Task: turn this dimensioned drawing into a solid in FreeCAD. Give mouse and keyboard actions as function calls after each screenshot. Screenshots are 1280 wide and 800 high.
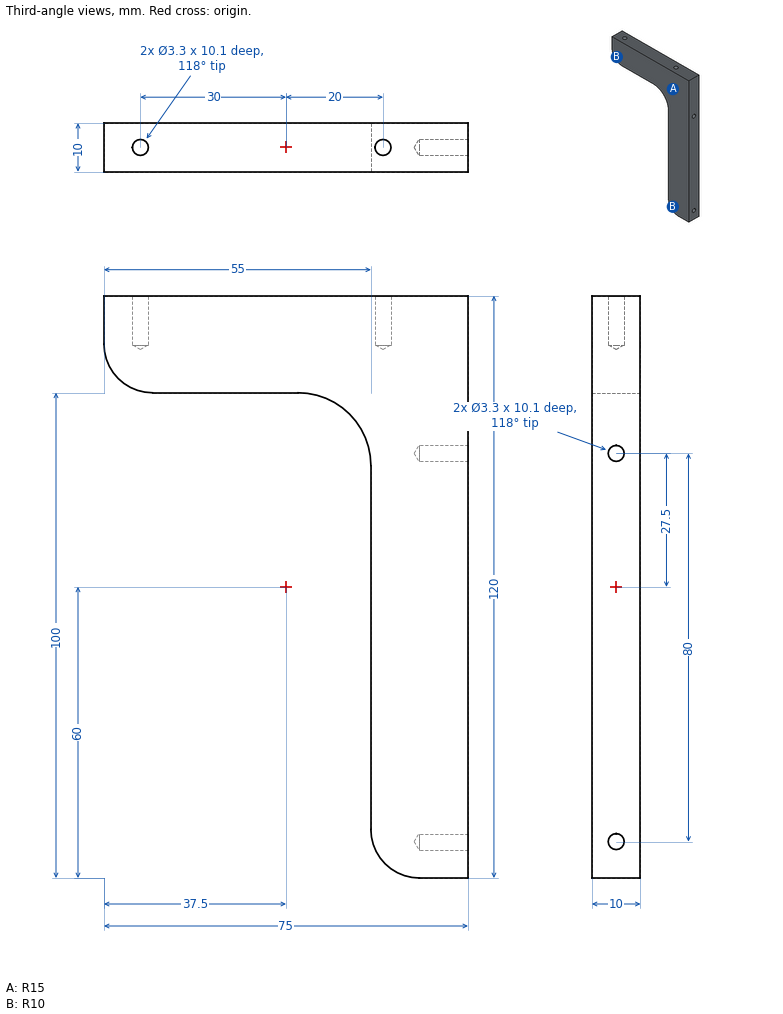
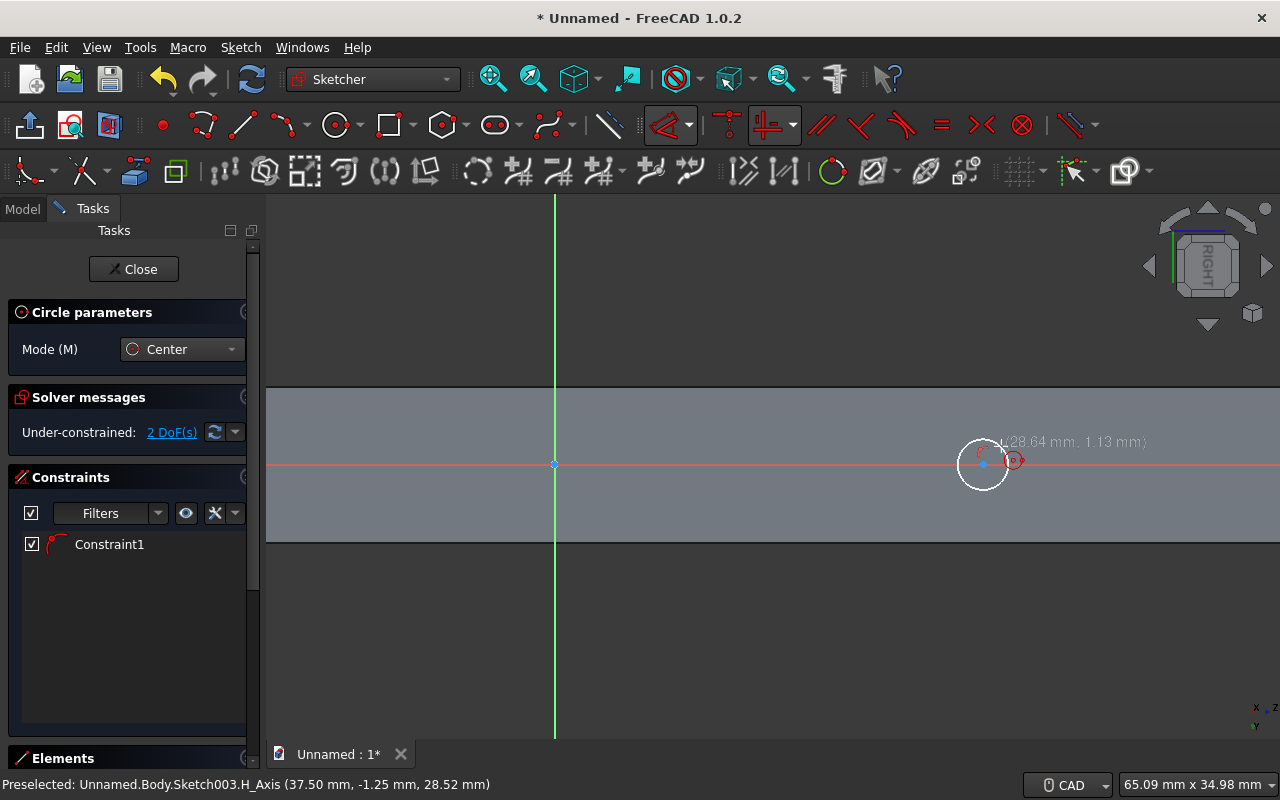
scroll(986, 468, down, 4)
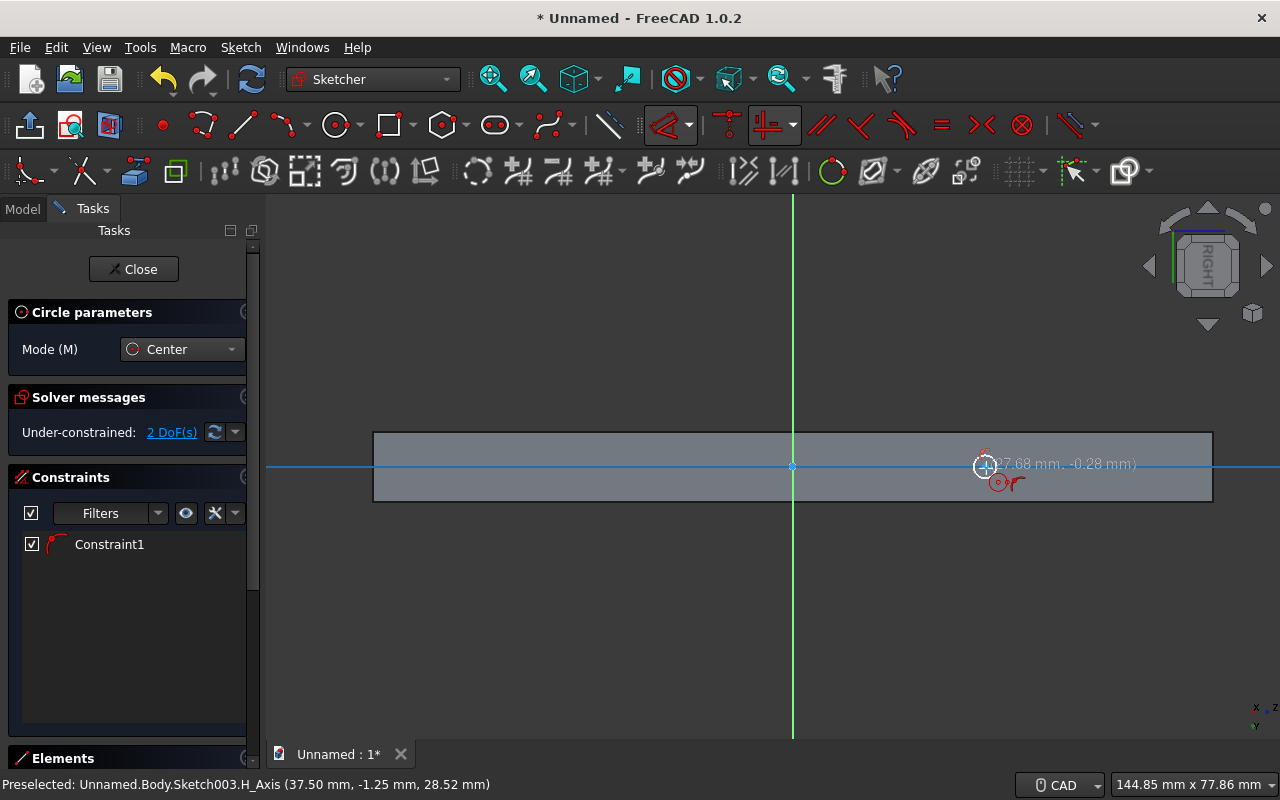
scroll(425, 467, up, 4)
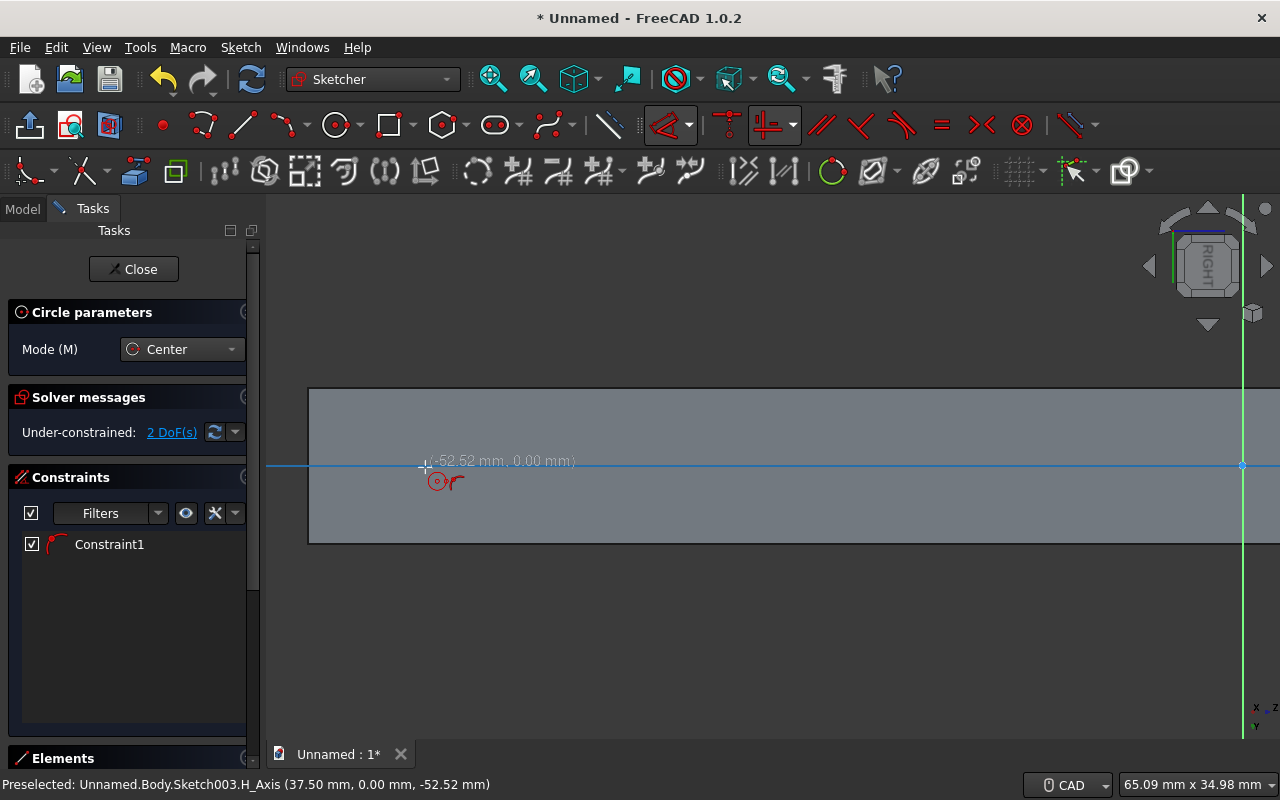
click(425, 466)
click(443, 448)
key(Escape)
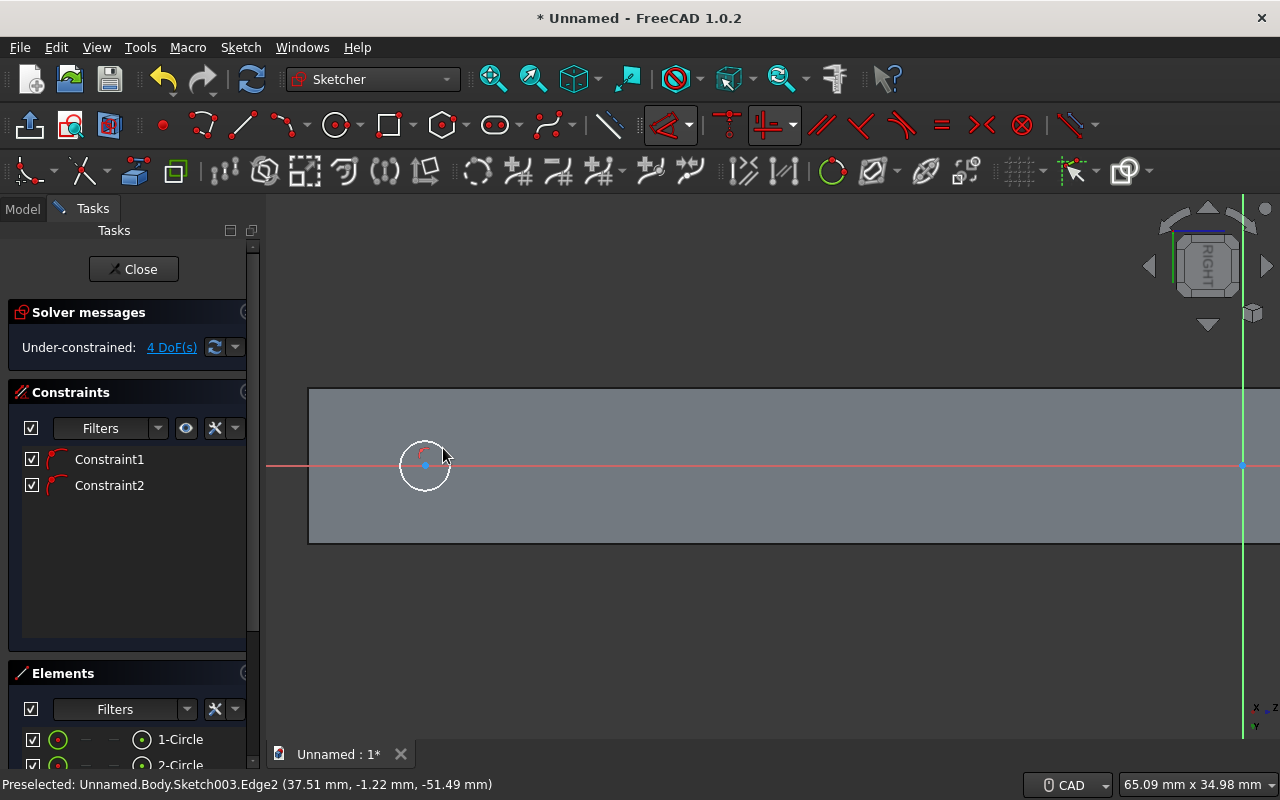
scroll(424, 467, down, 4)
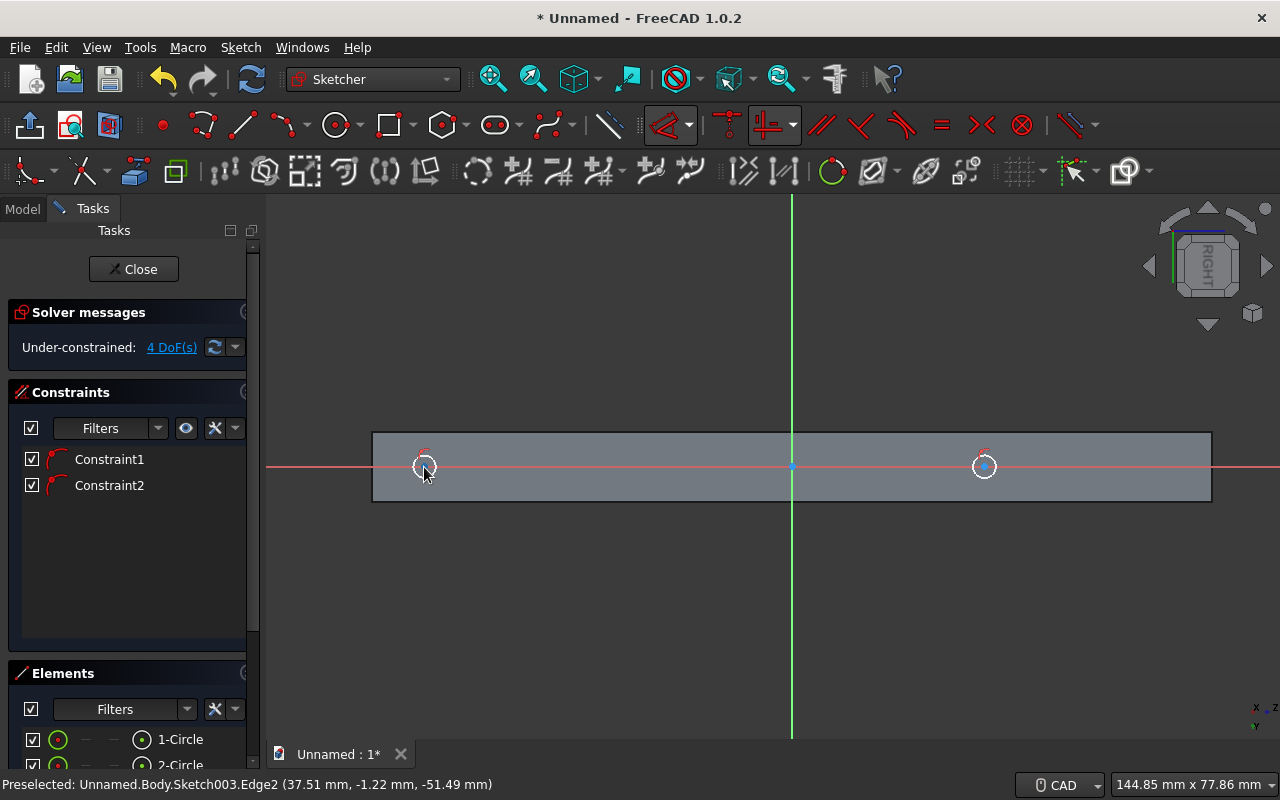
scroll(992, 459, up, 3)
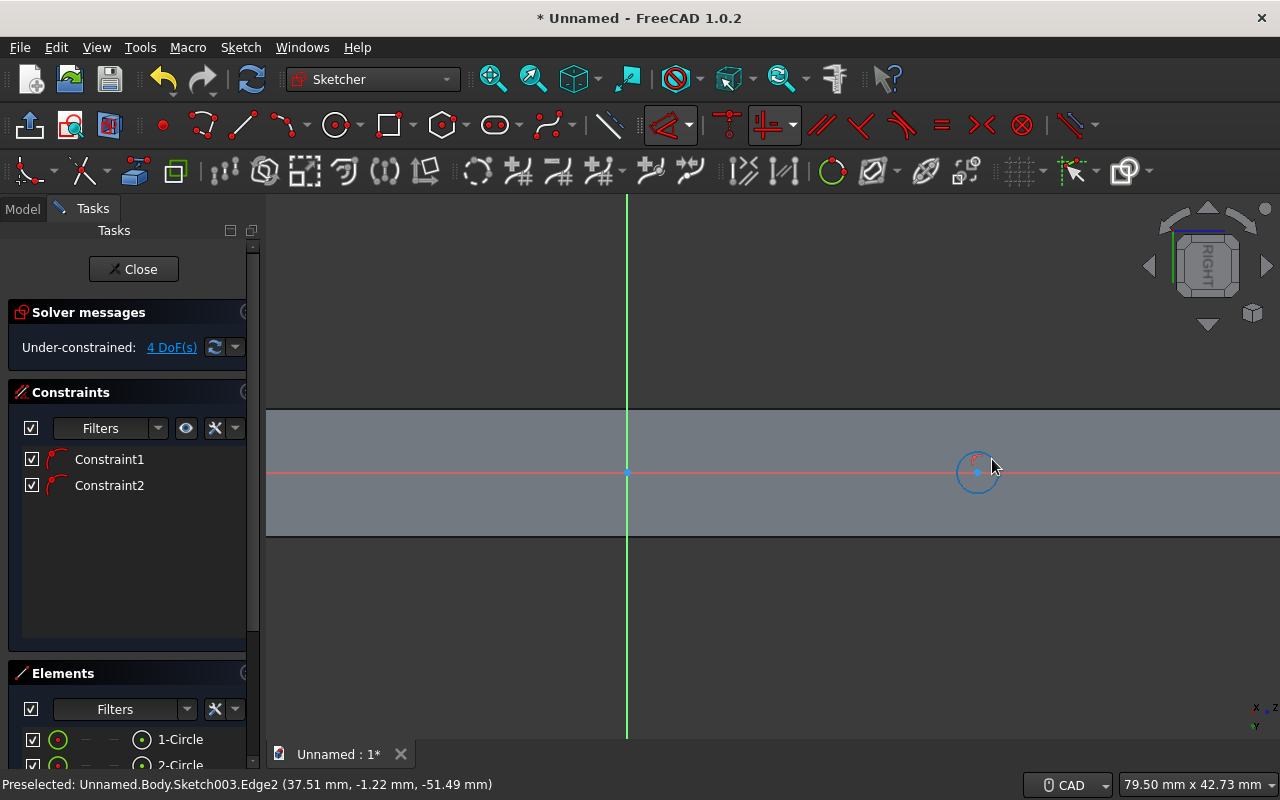
click(992, 458)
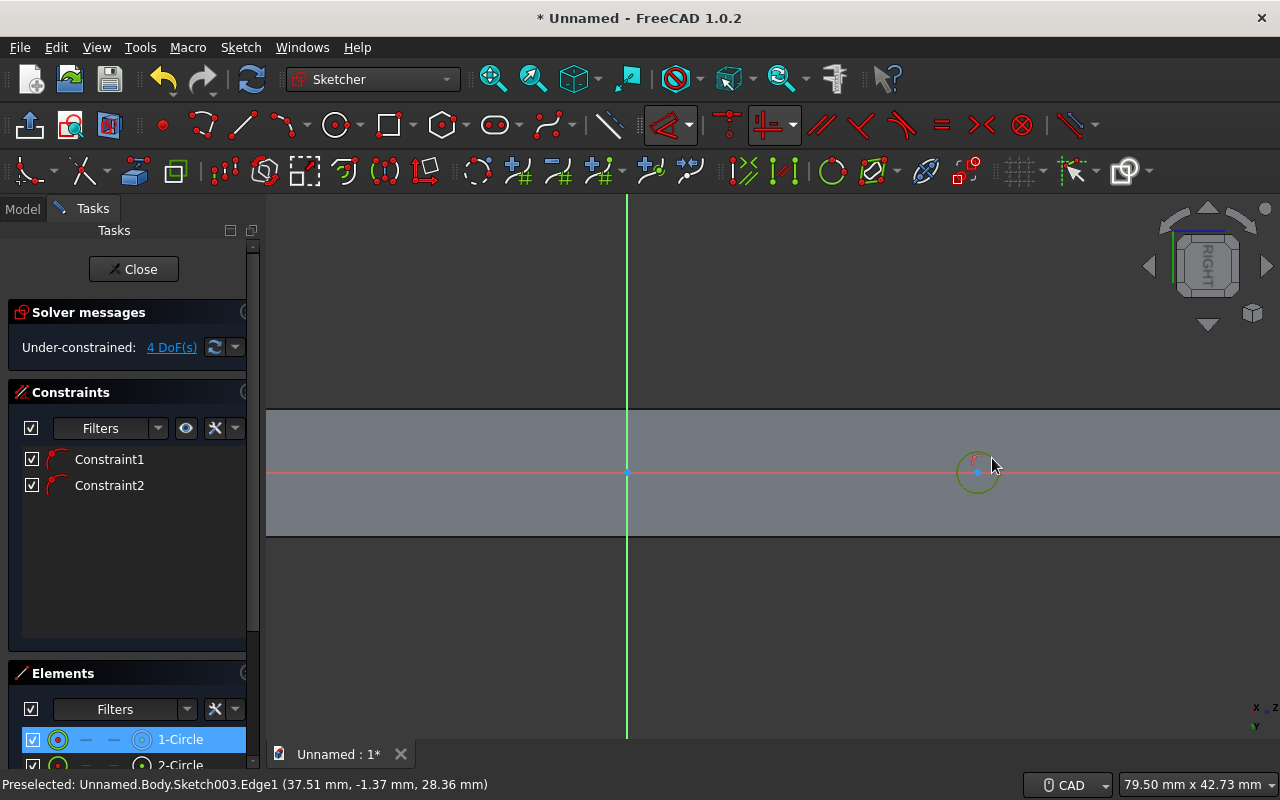
scroll(993, 459, down, 3)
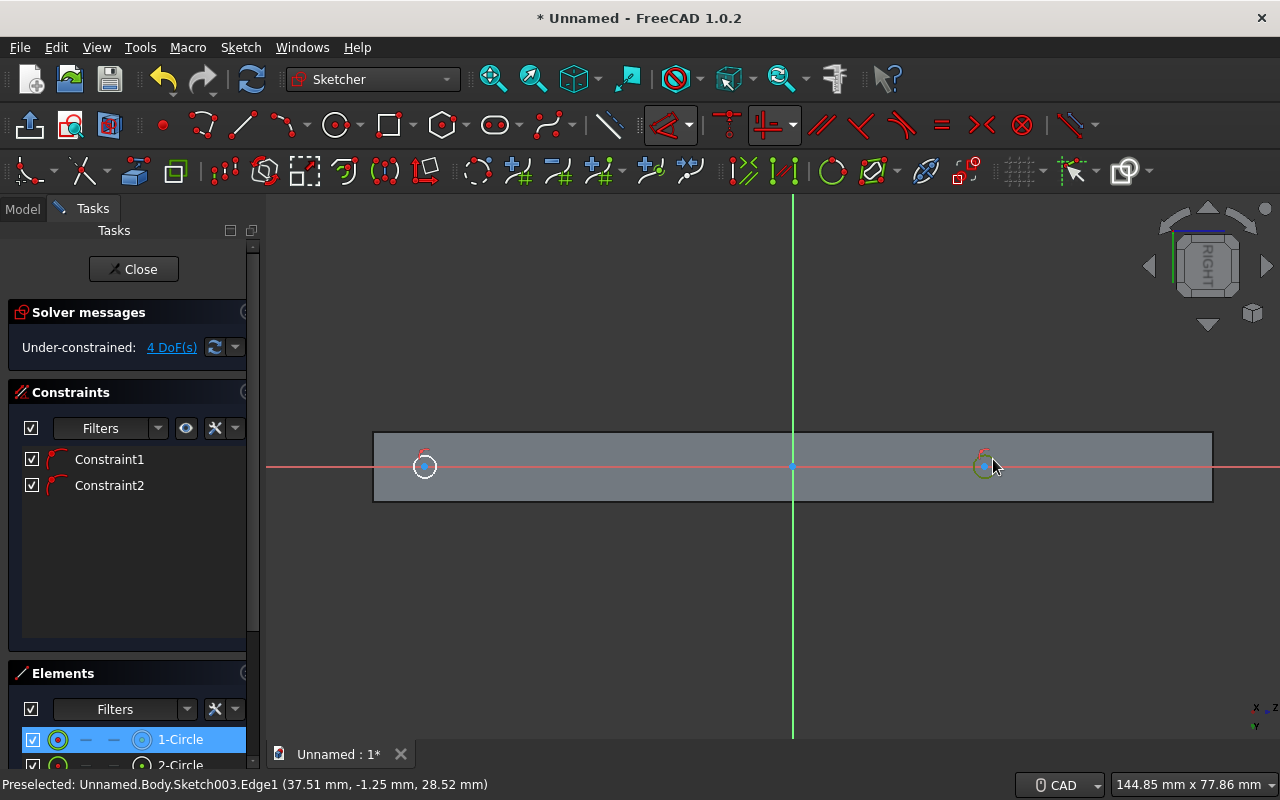
scroll(433, 459, up, 3)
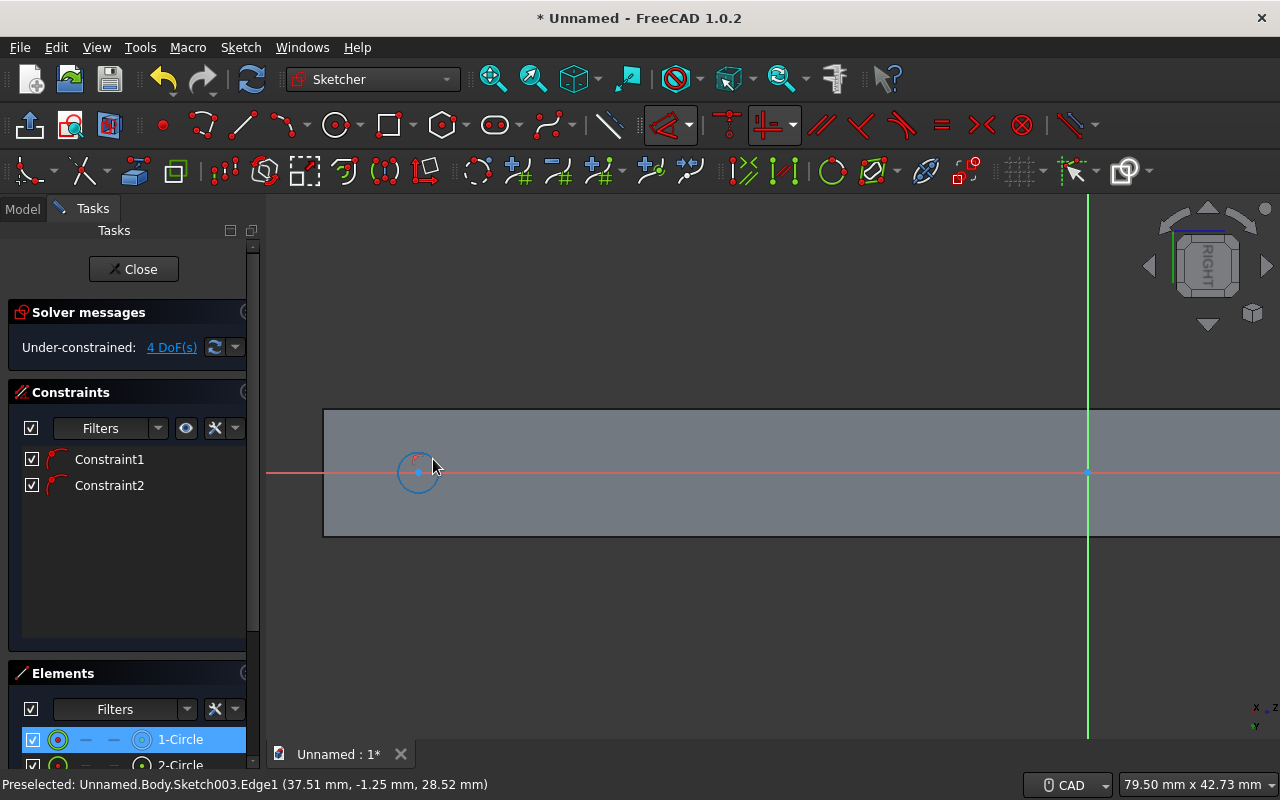
click(433, 458)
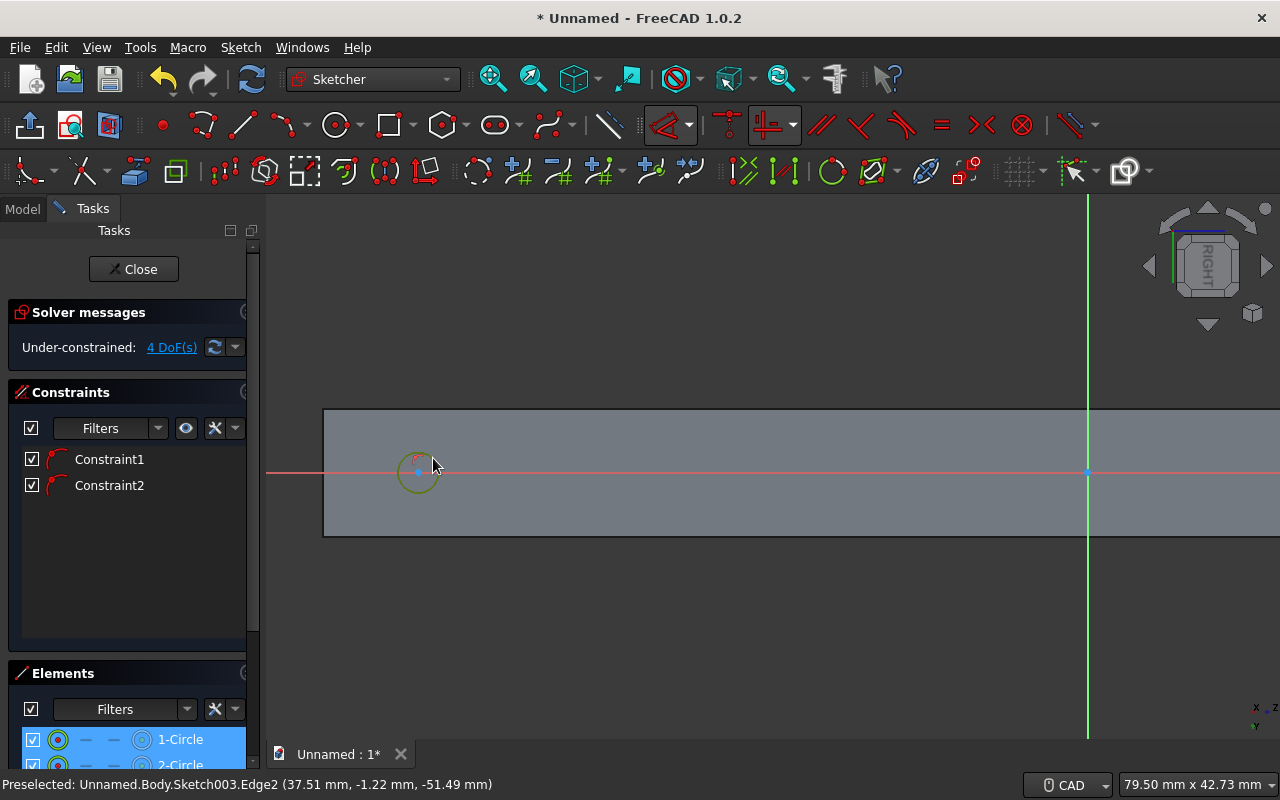
key(e)